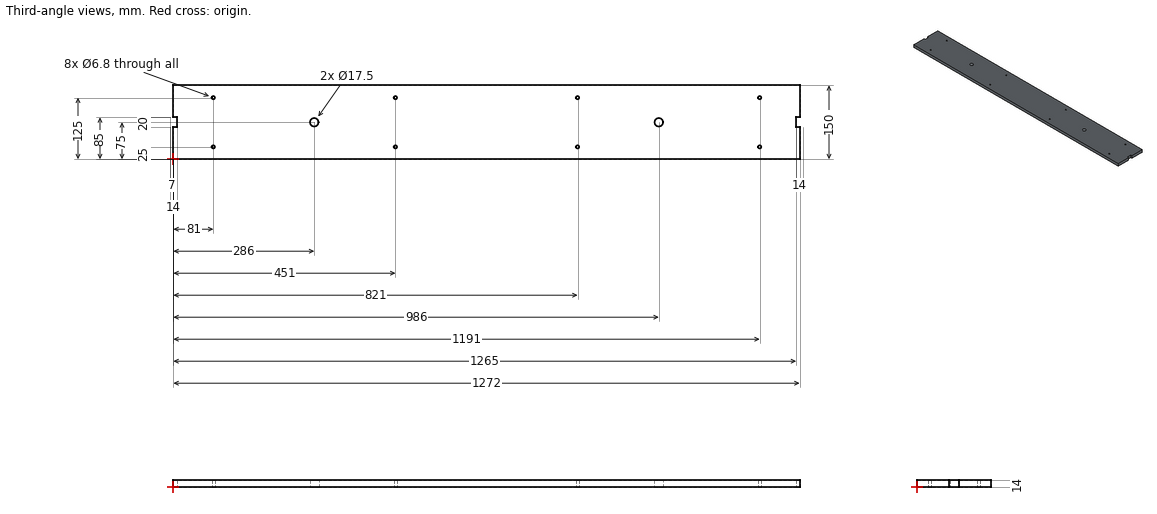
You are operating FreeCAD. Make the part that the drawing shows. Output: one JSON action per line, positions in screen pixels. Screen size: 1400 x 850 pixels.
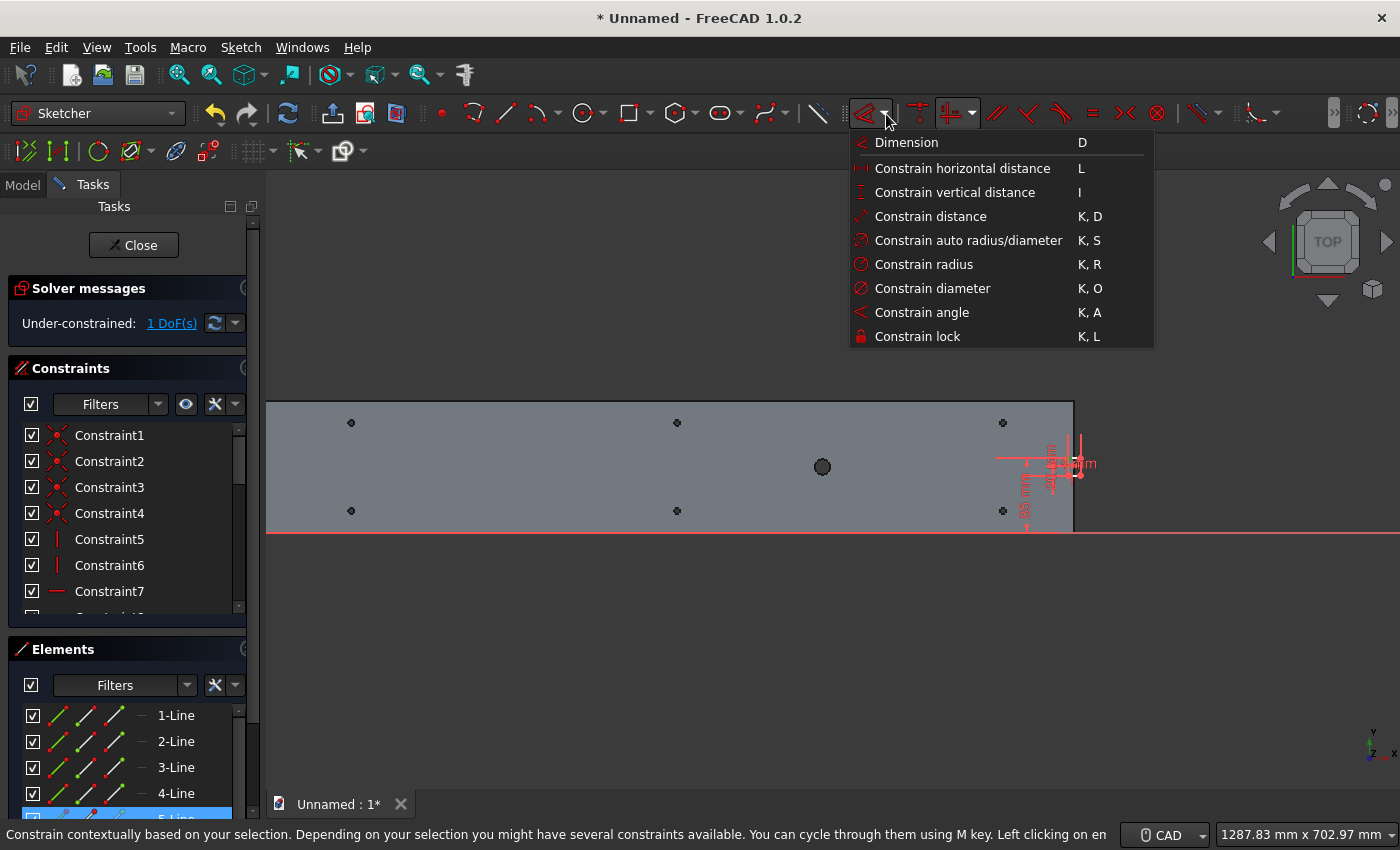
{"action": "left_click", "coordinate": [1002, 168]}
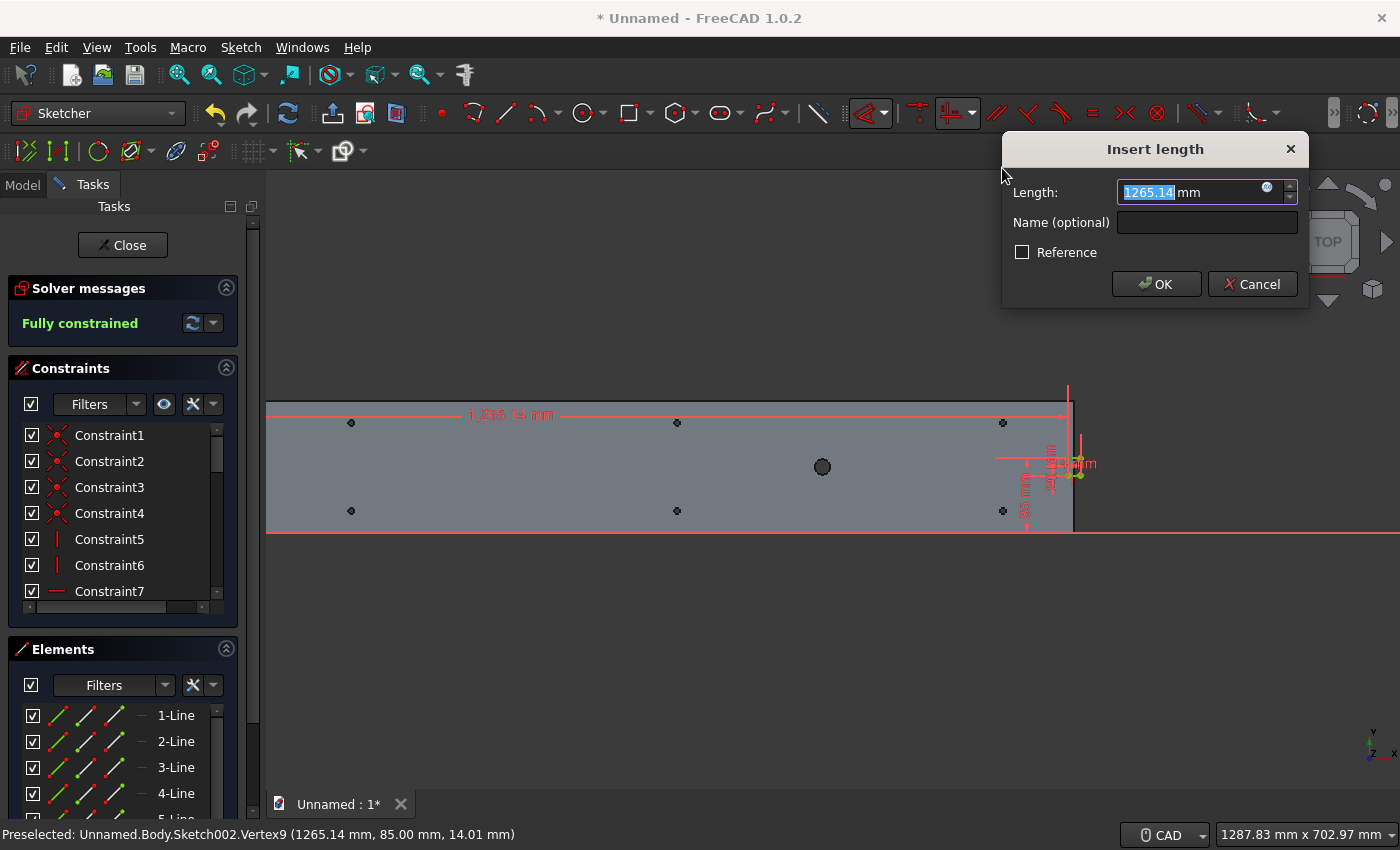
{"action": "type", "text": "1265"}
{"action": "key", "text": "Return"}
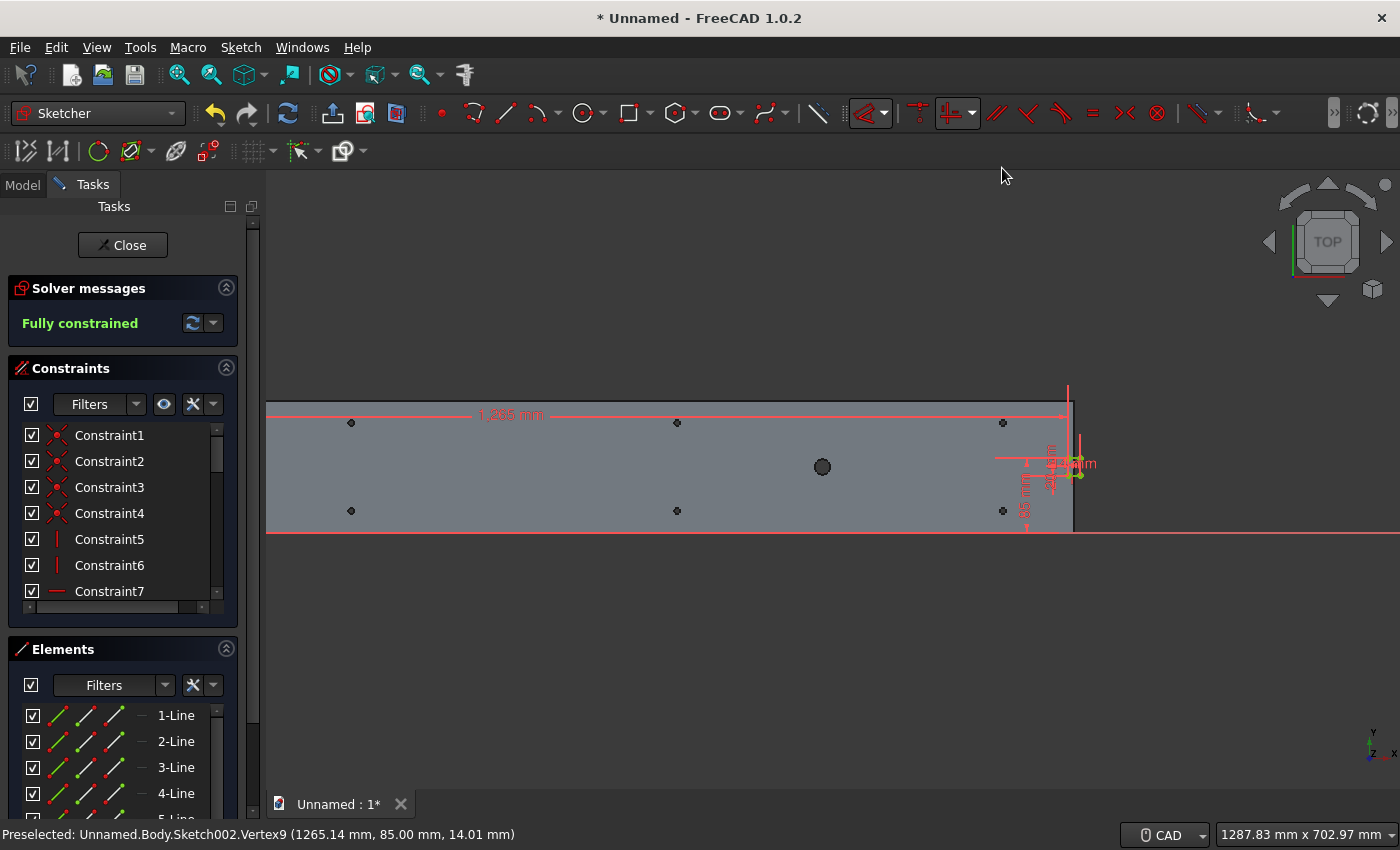
{"action": "left_click", "coordinate": [123, 245]}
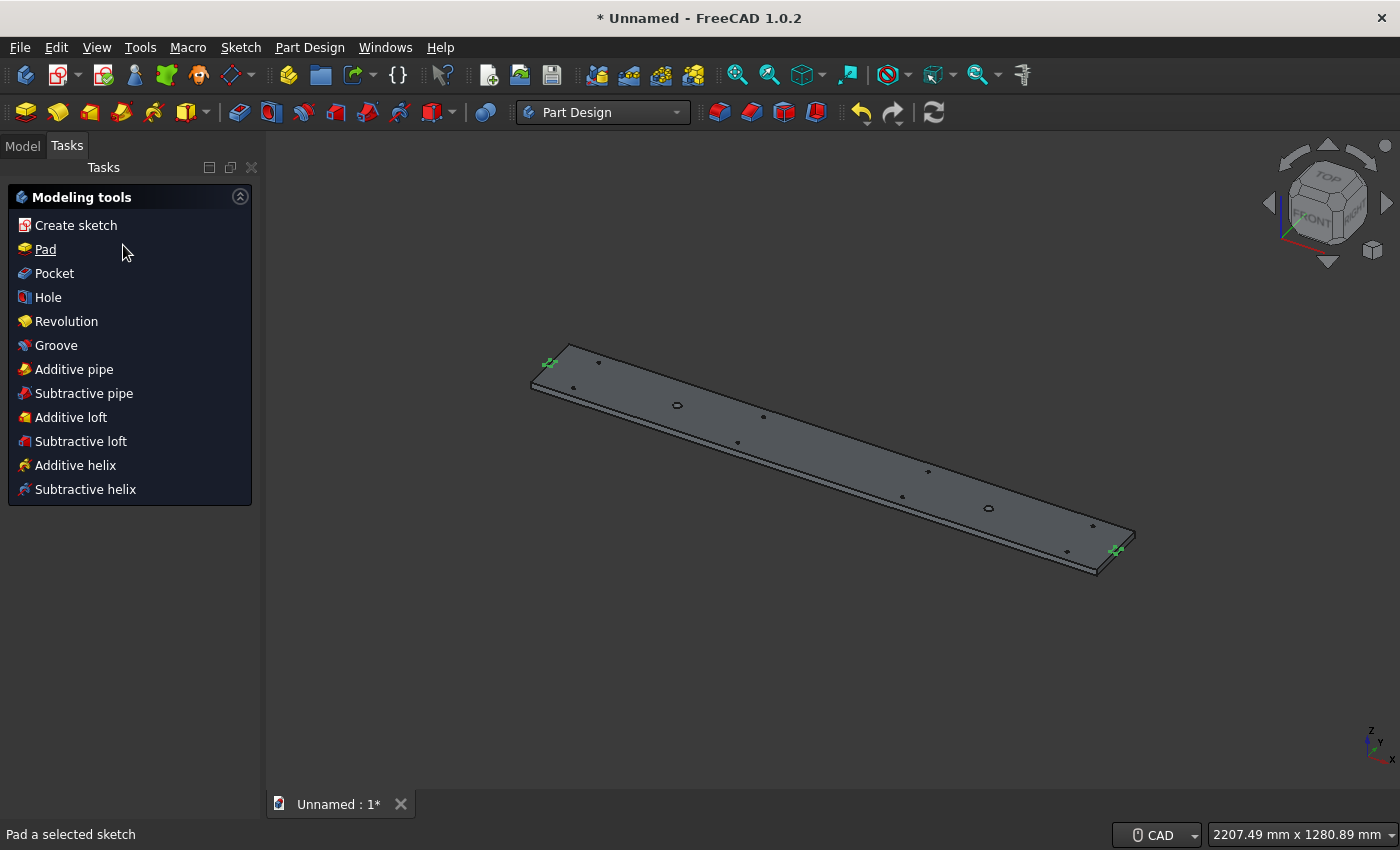
{"action": "left_click", "coordinate": [240, 112]}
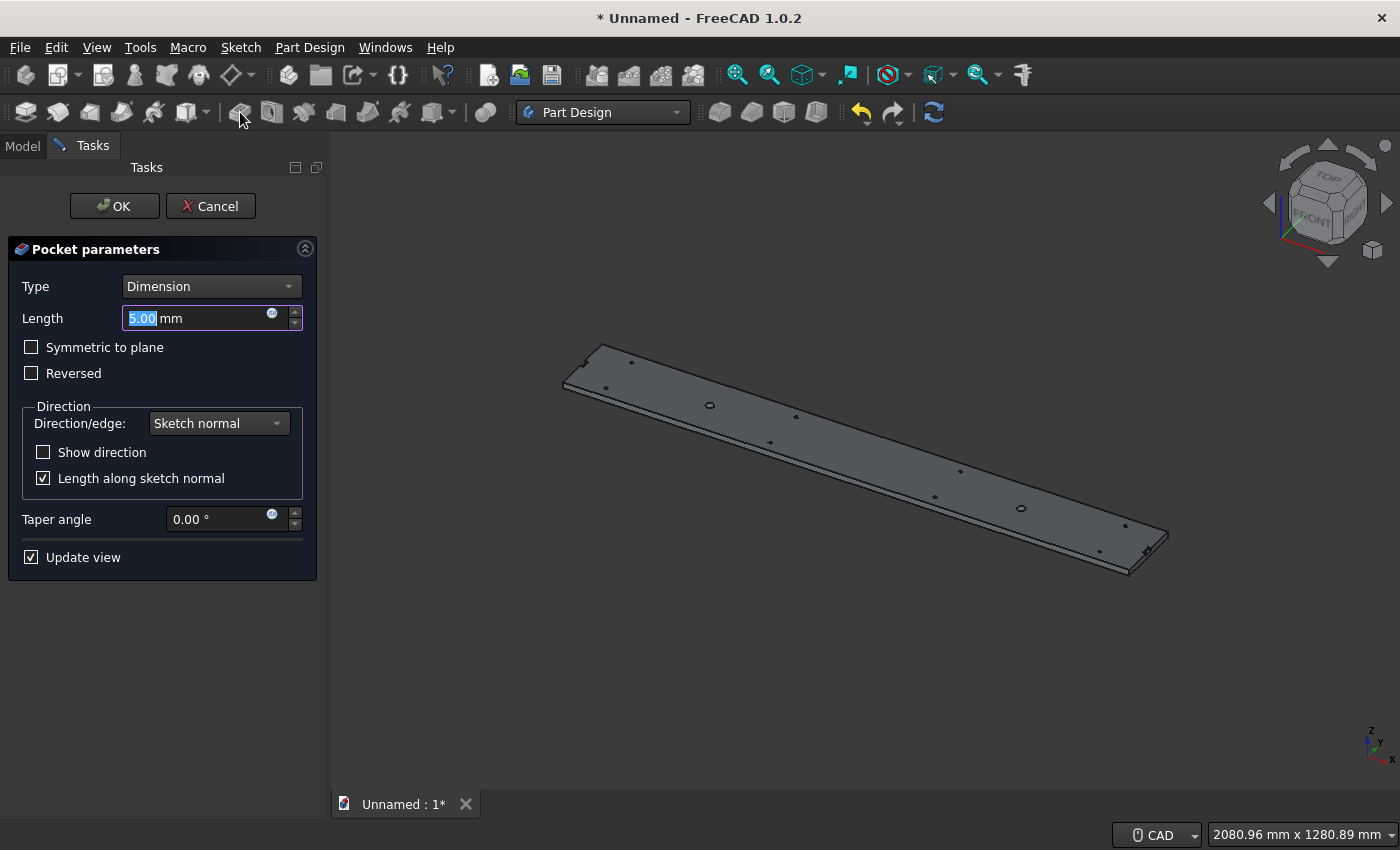
{"action": "left_click", "coordinate": [212, 286]}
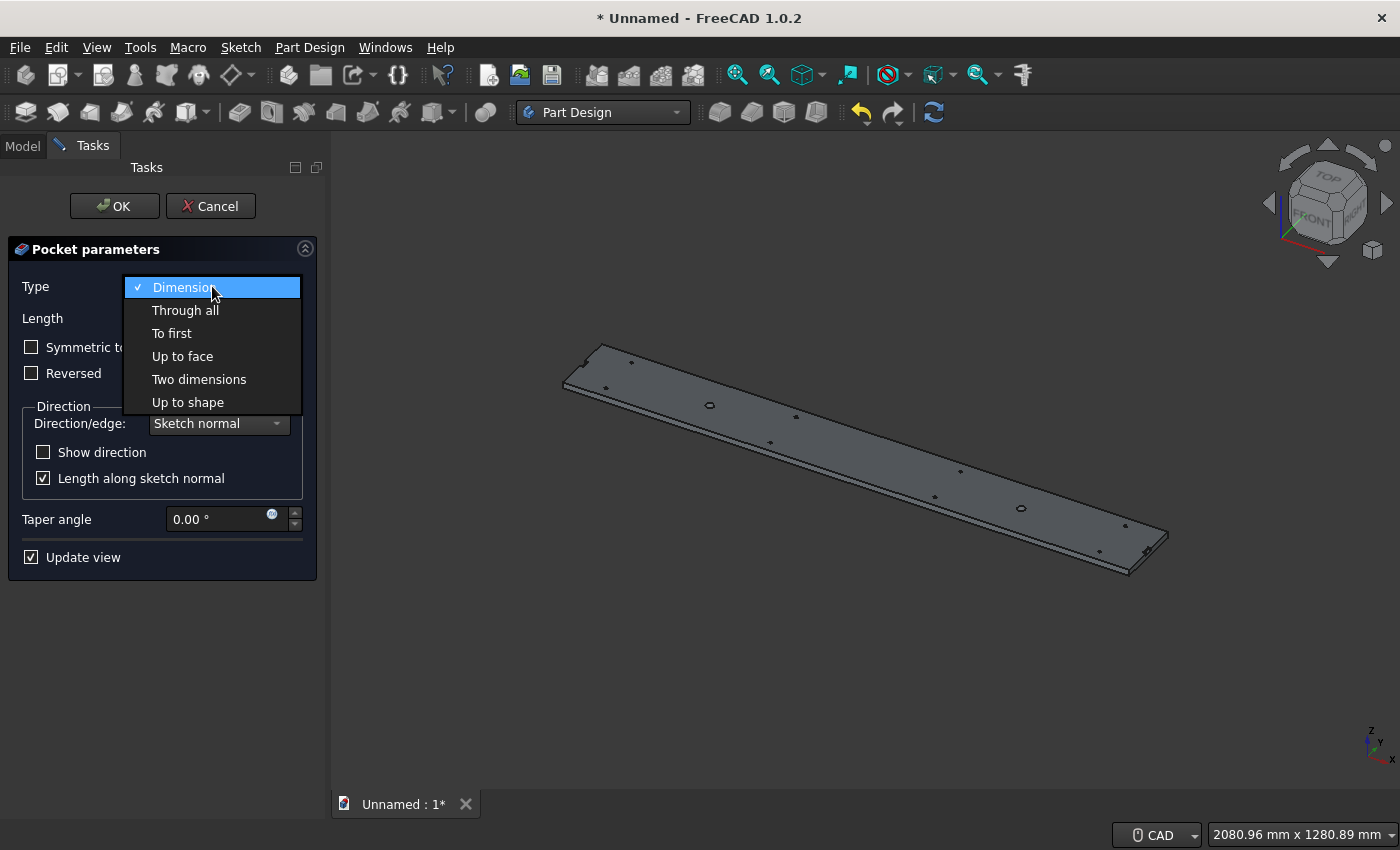
{"action": "left_click", "coordinate": [212, 310]}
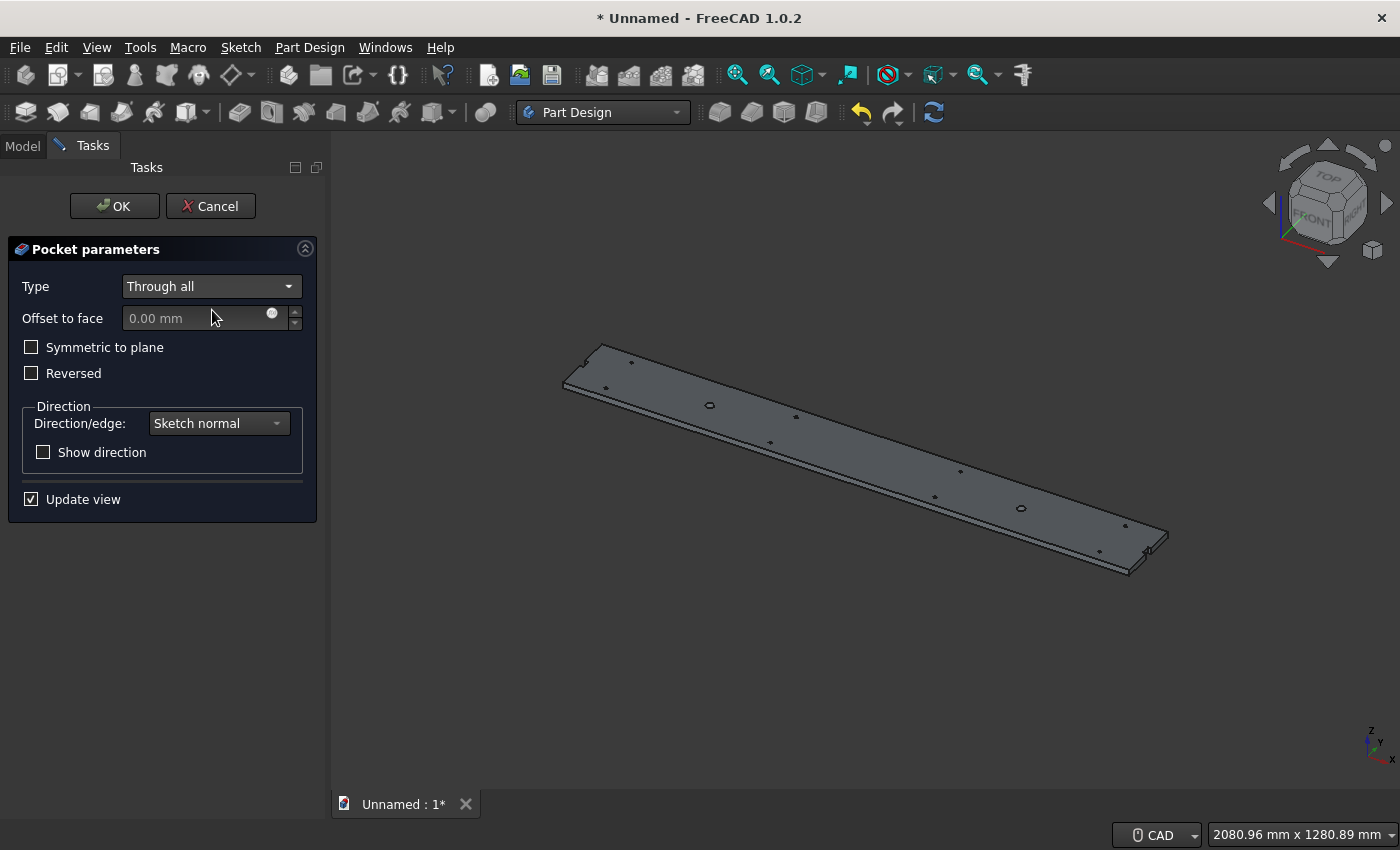
{"action": "left_click", "coordinate": [115, 206]}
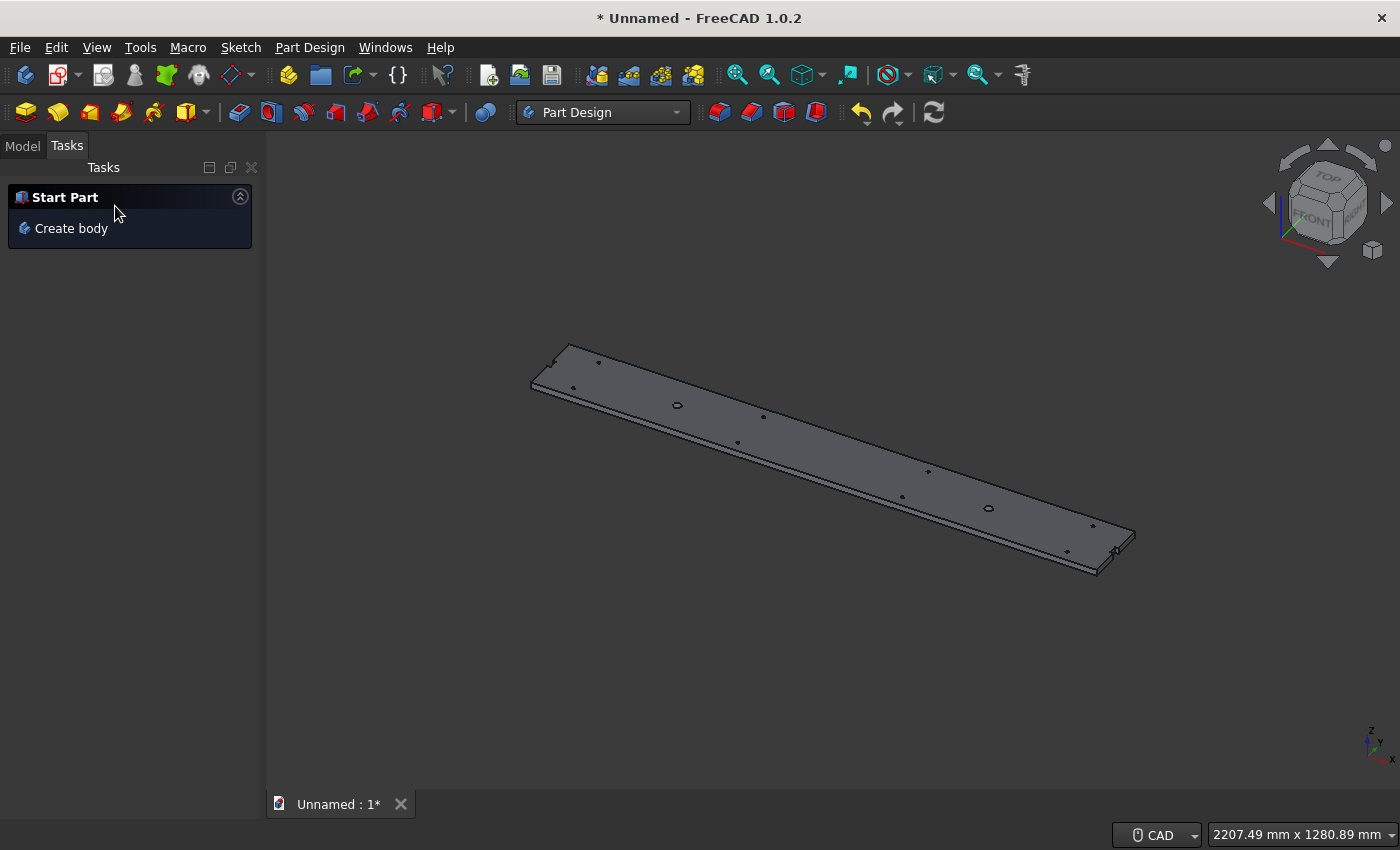
{"action": "key", "text": "0"}